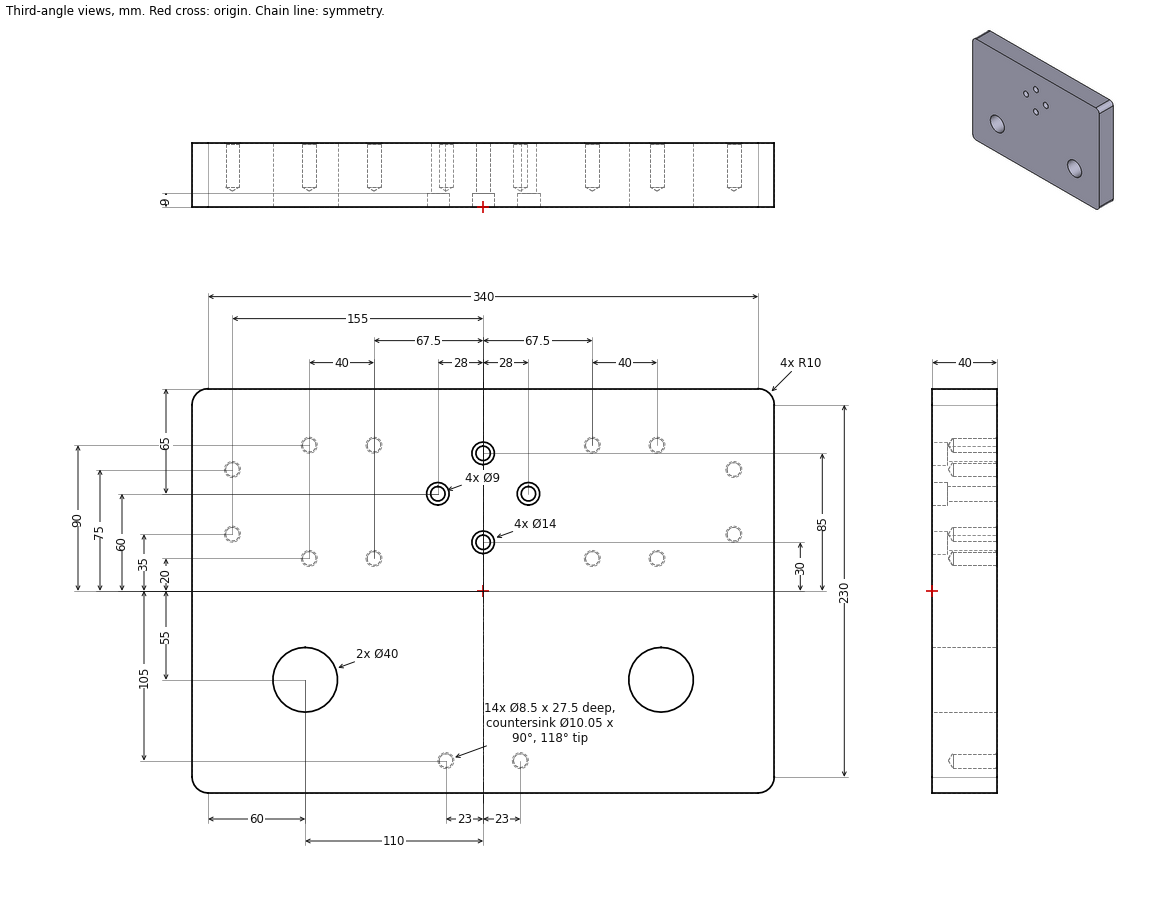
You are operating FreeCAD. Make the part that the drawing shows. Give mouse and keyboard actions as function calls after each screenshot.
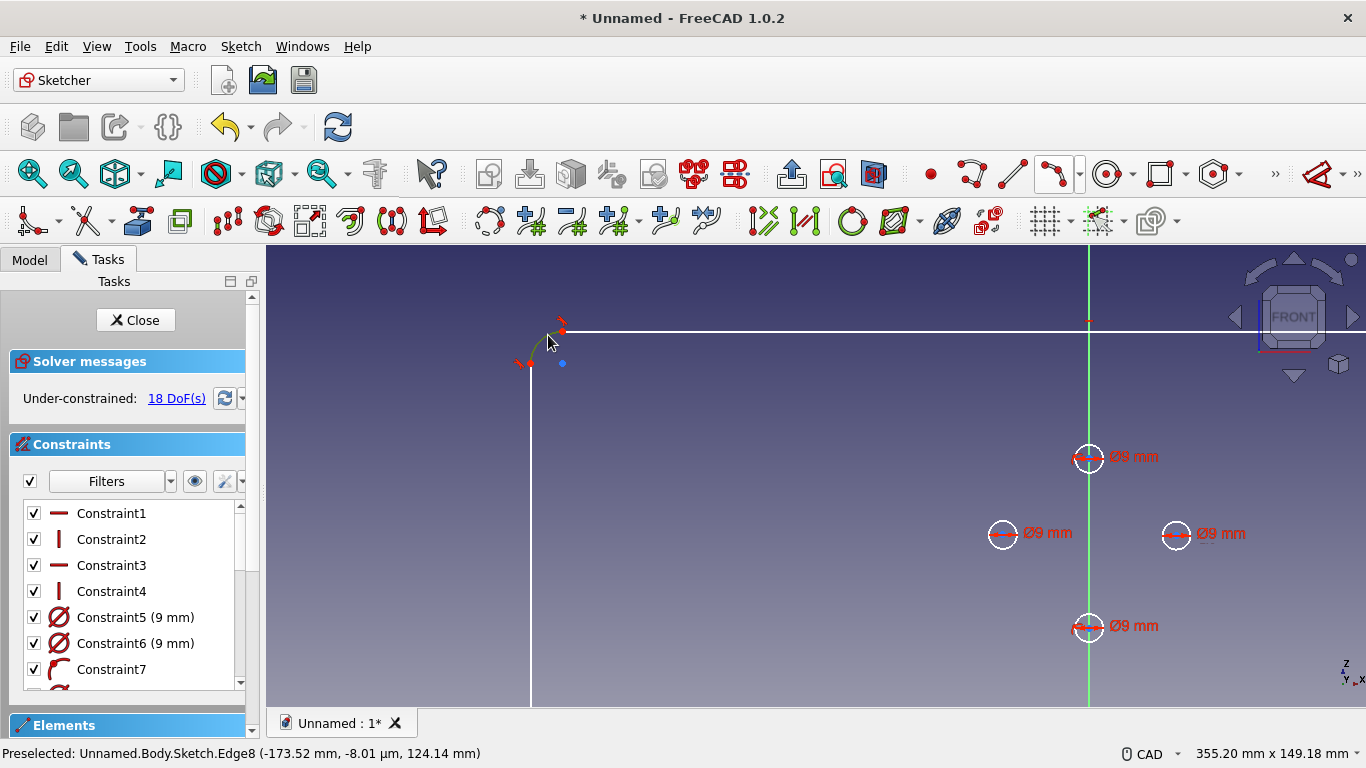
key(e)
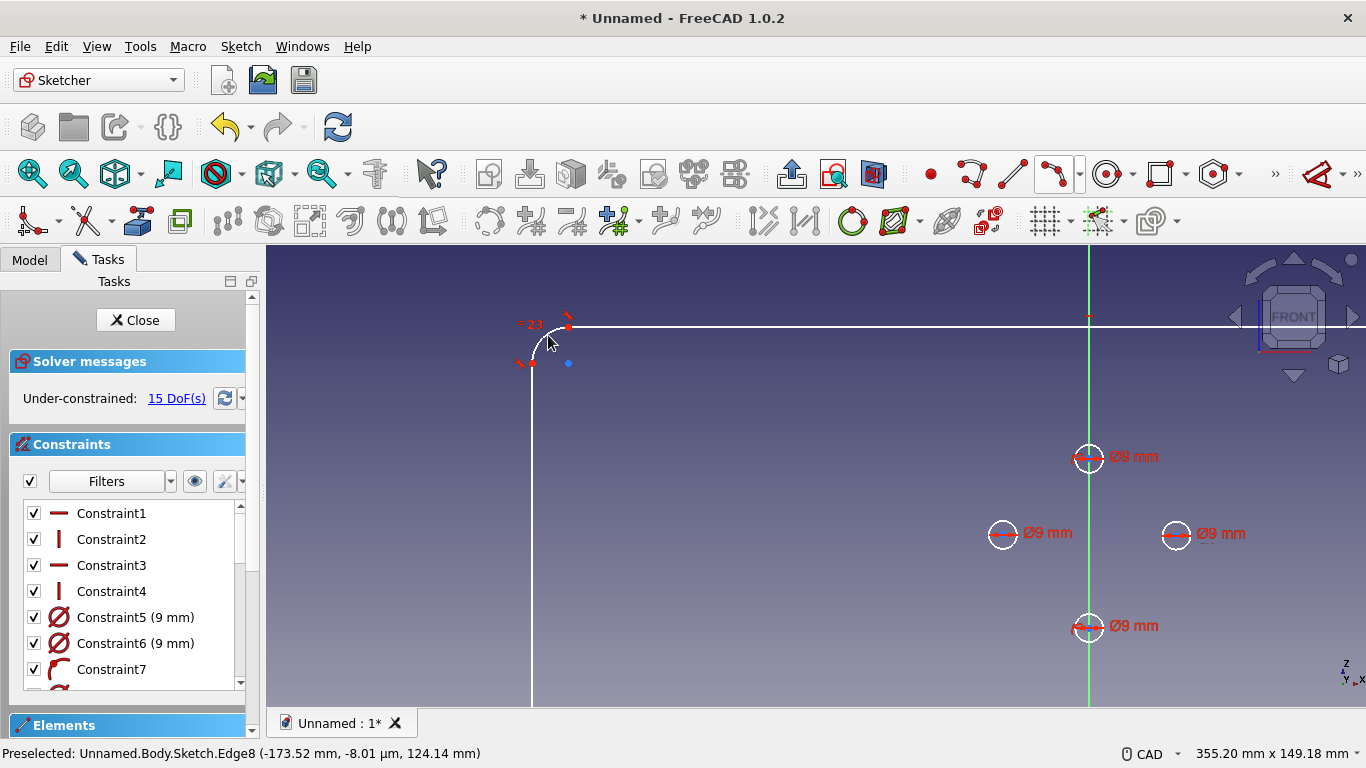
click(1003, 535)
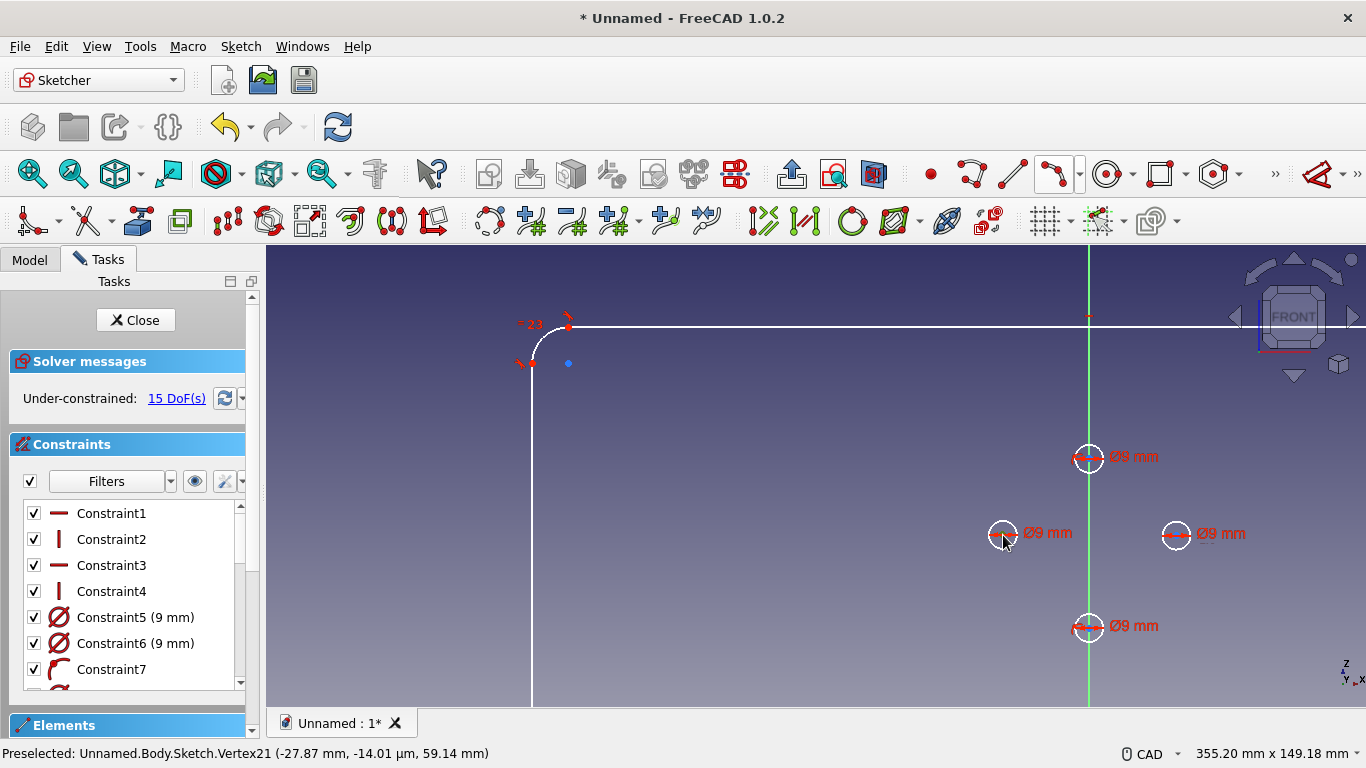
click(1176, 536)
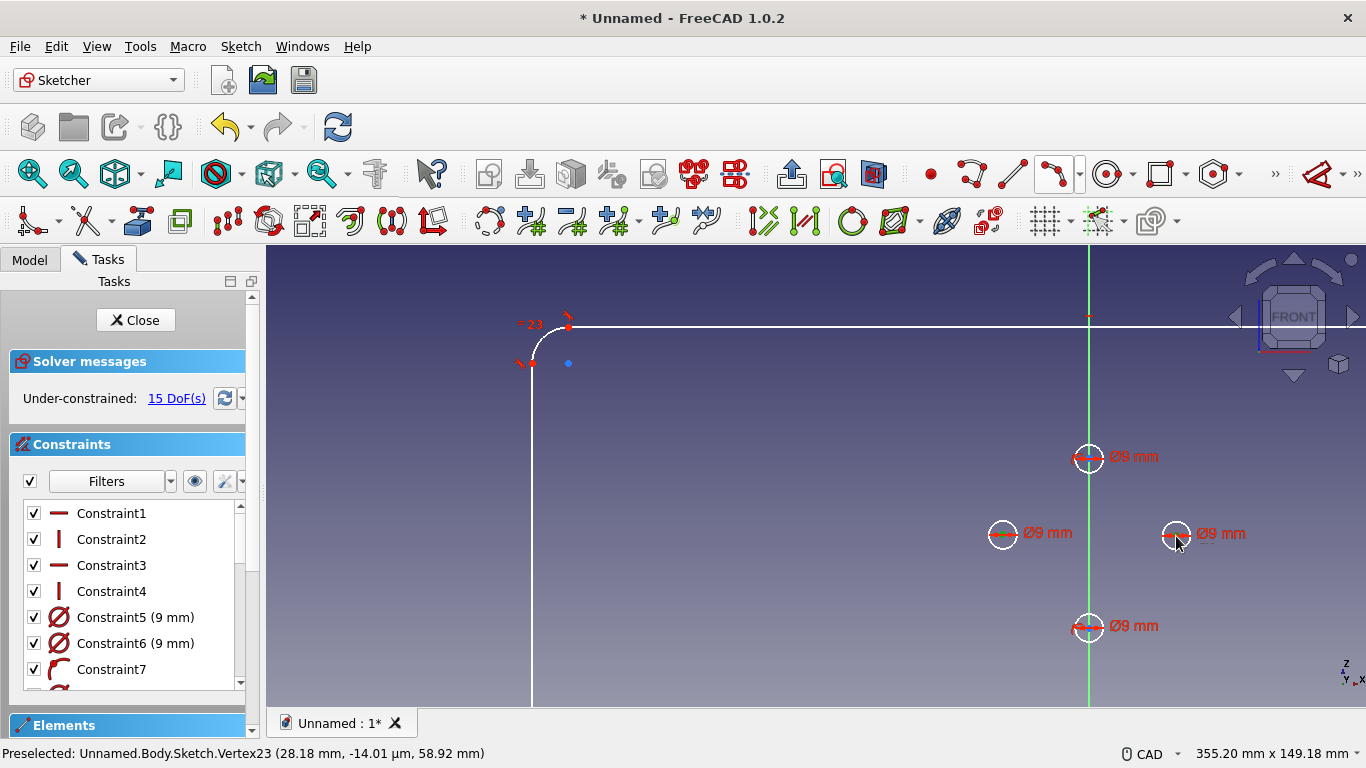
key(h)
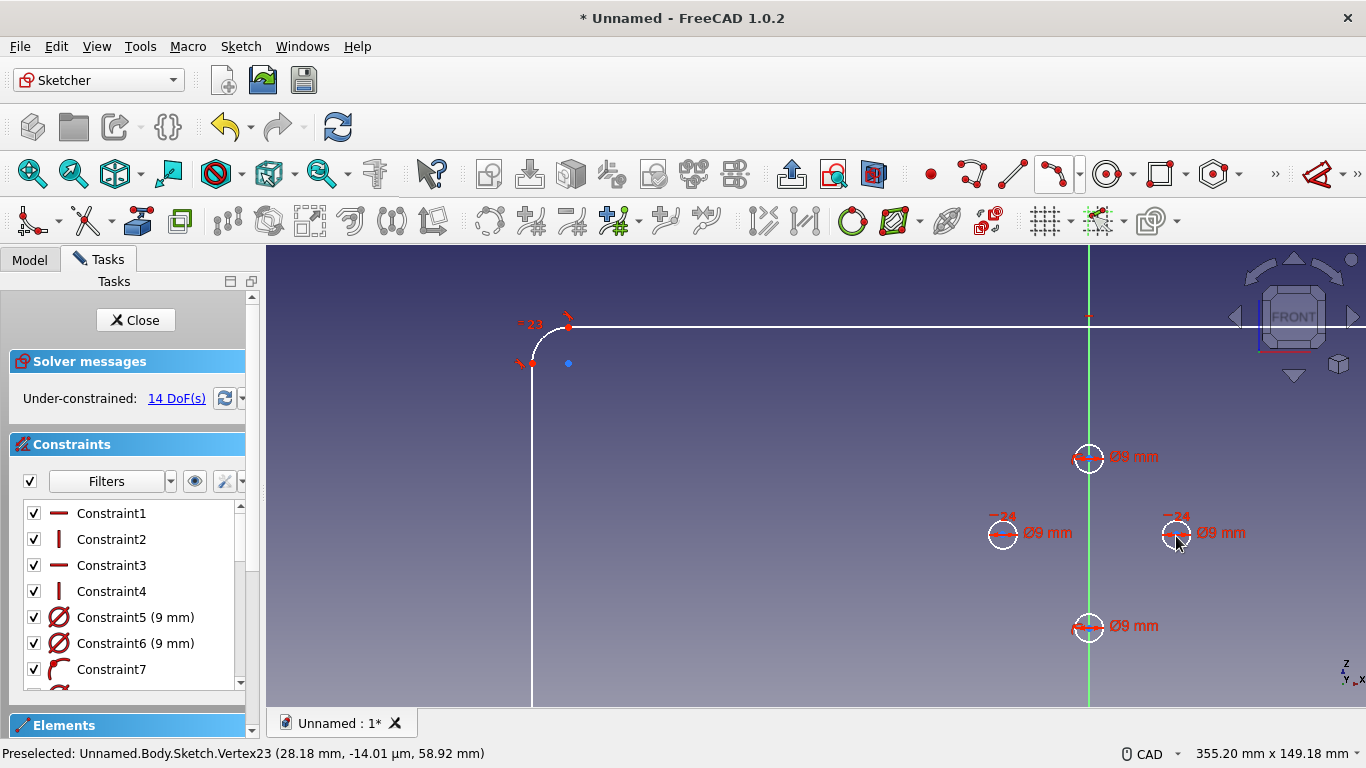
scroll(549, 335, down, 5)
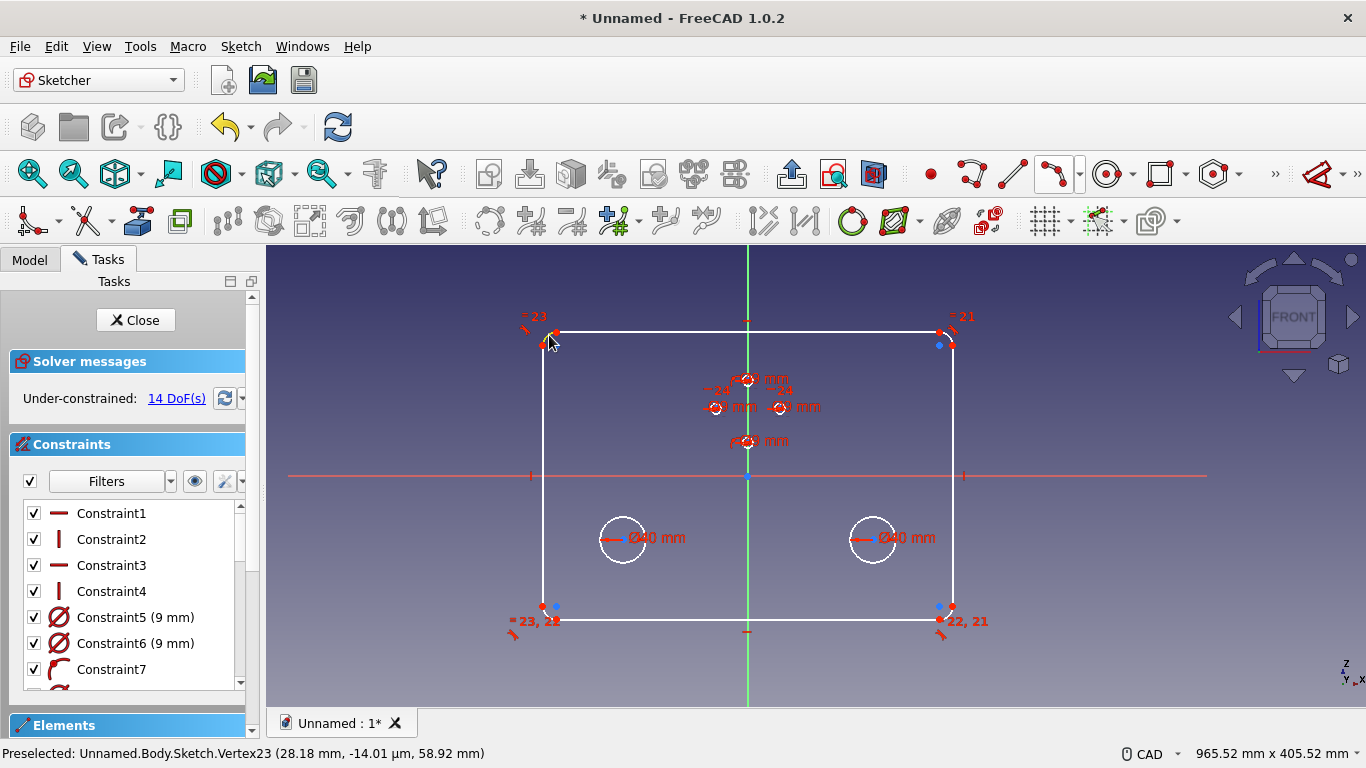
click(623, 540)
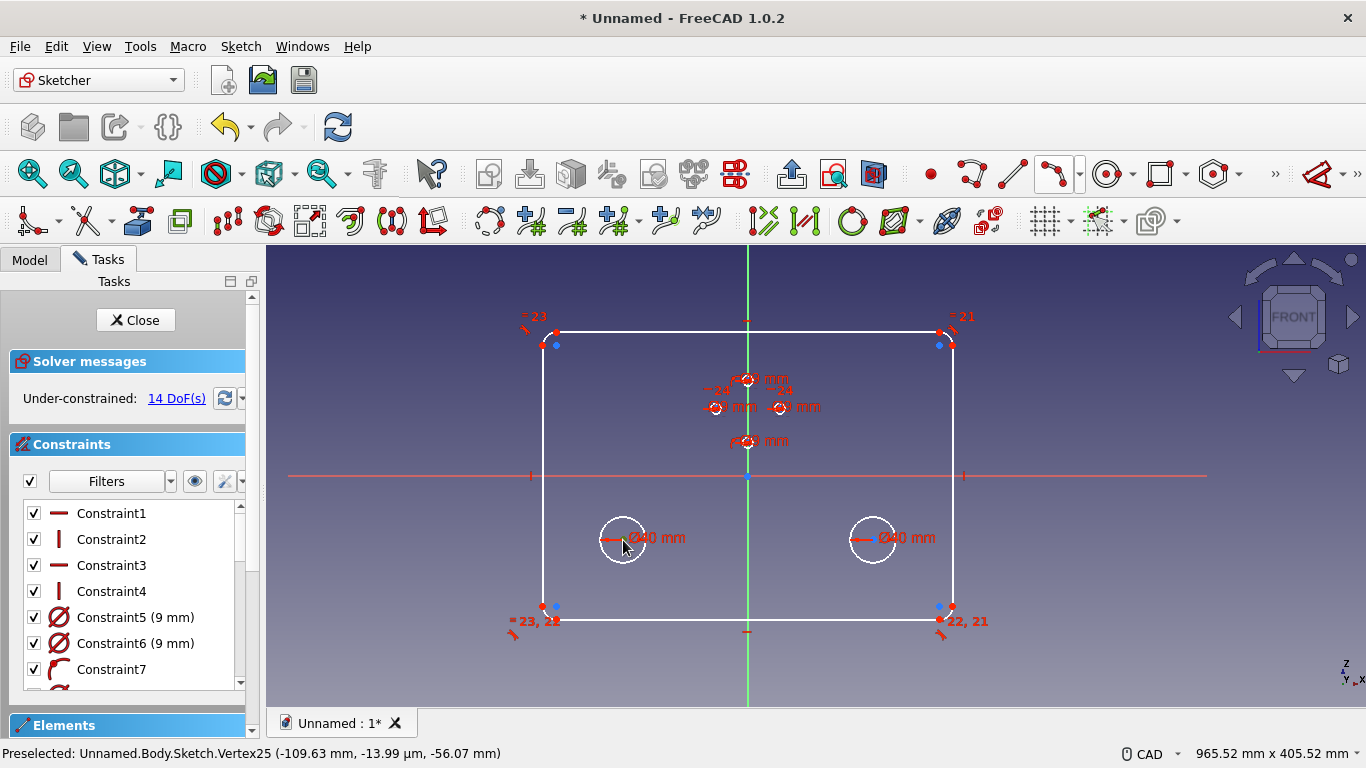
click(873, 540)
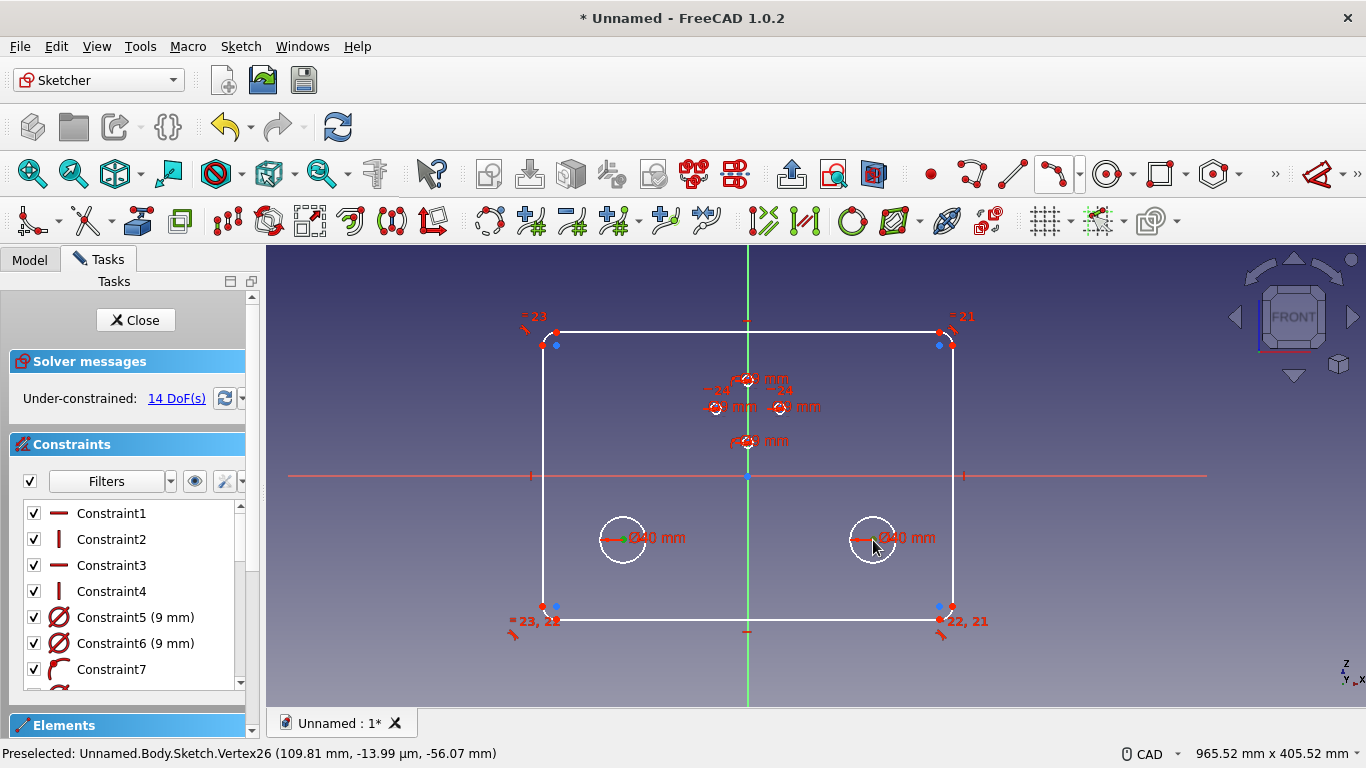
click(748, 650)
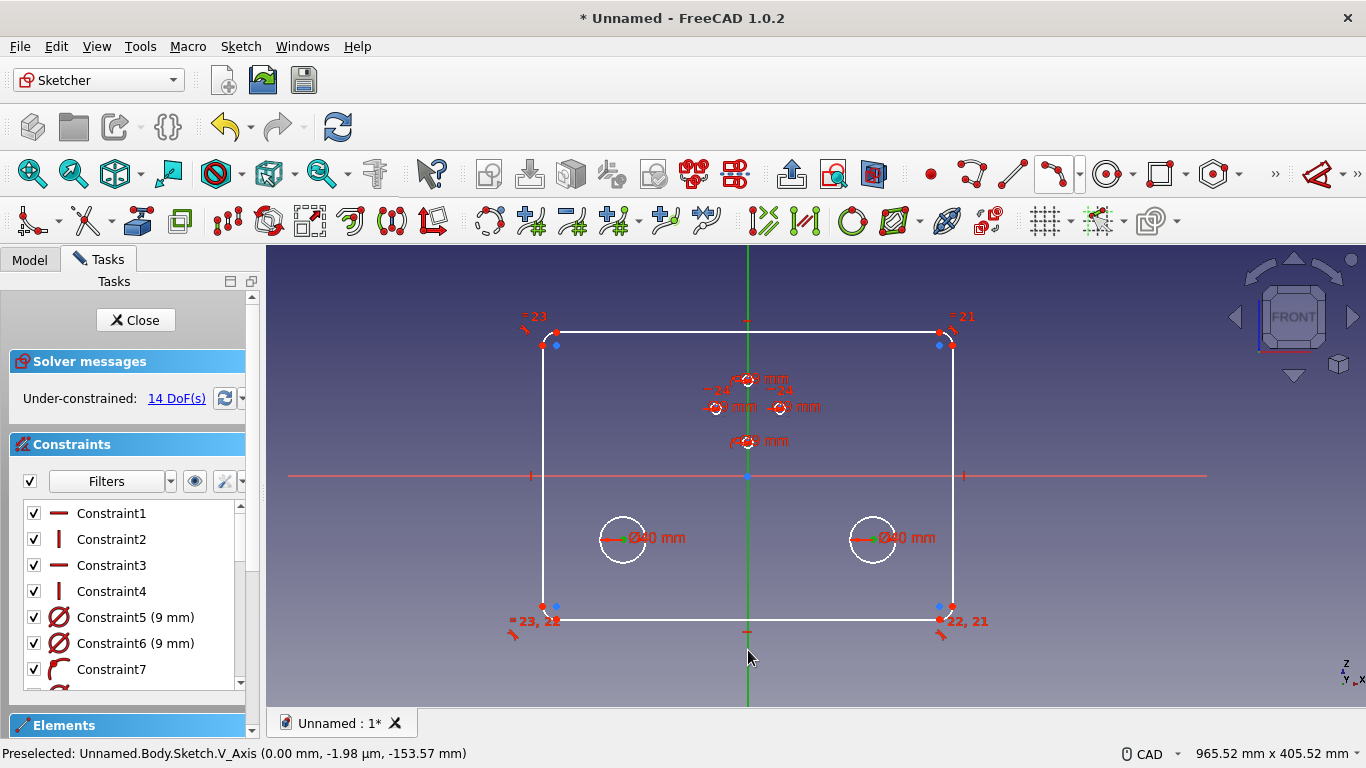
key(s)